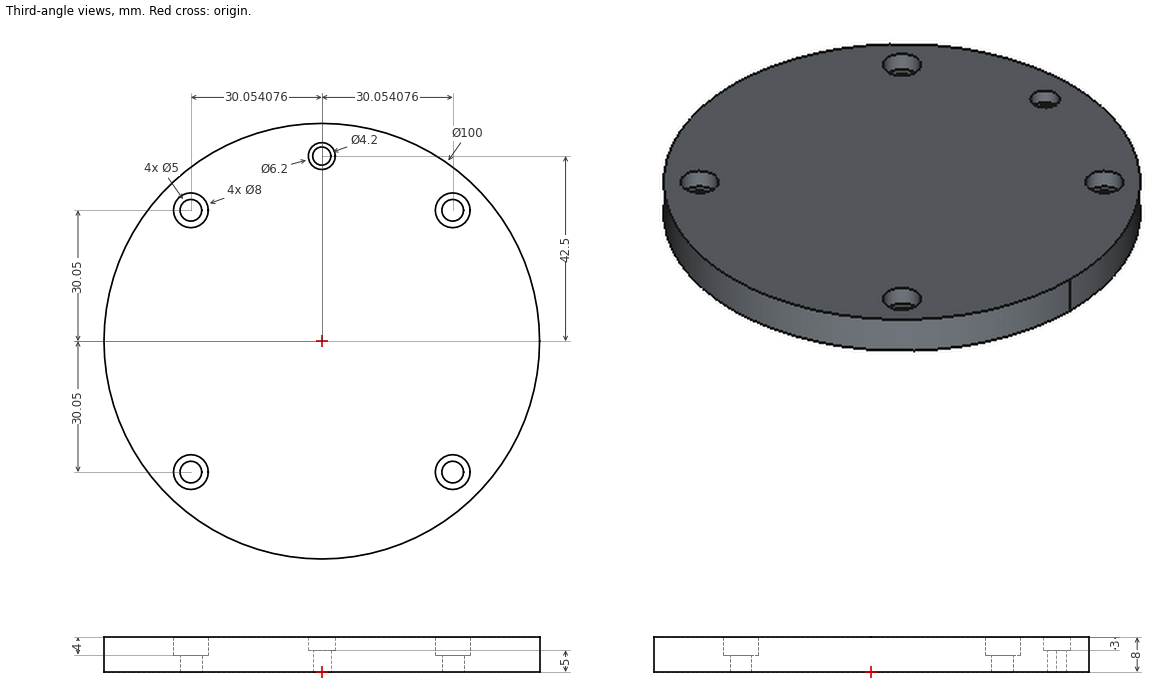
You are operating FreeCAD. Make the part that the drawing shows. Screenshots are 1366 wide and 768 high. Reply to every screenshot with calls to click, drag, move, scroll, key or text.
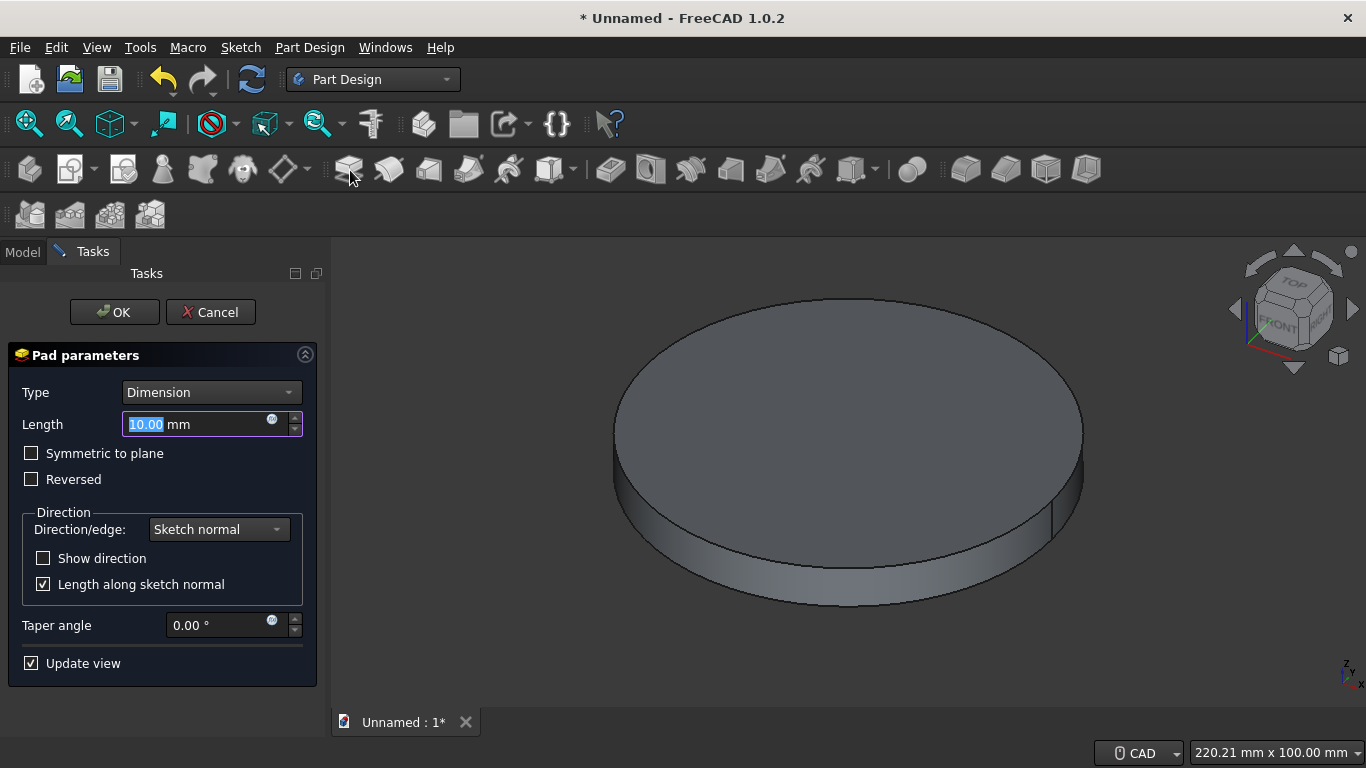
text(8)
key(Tab)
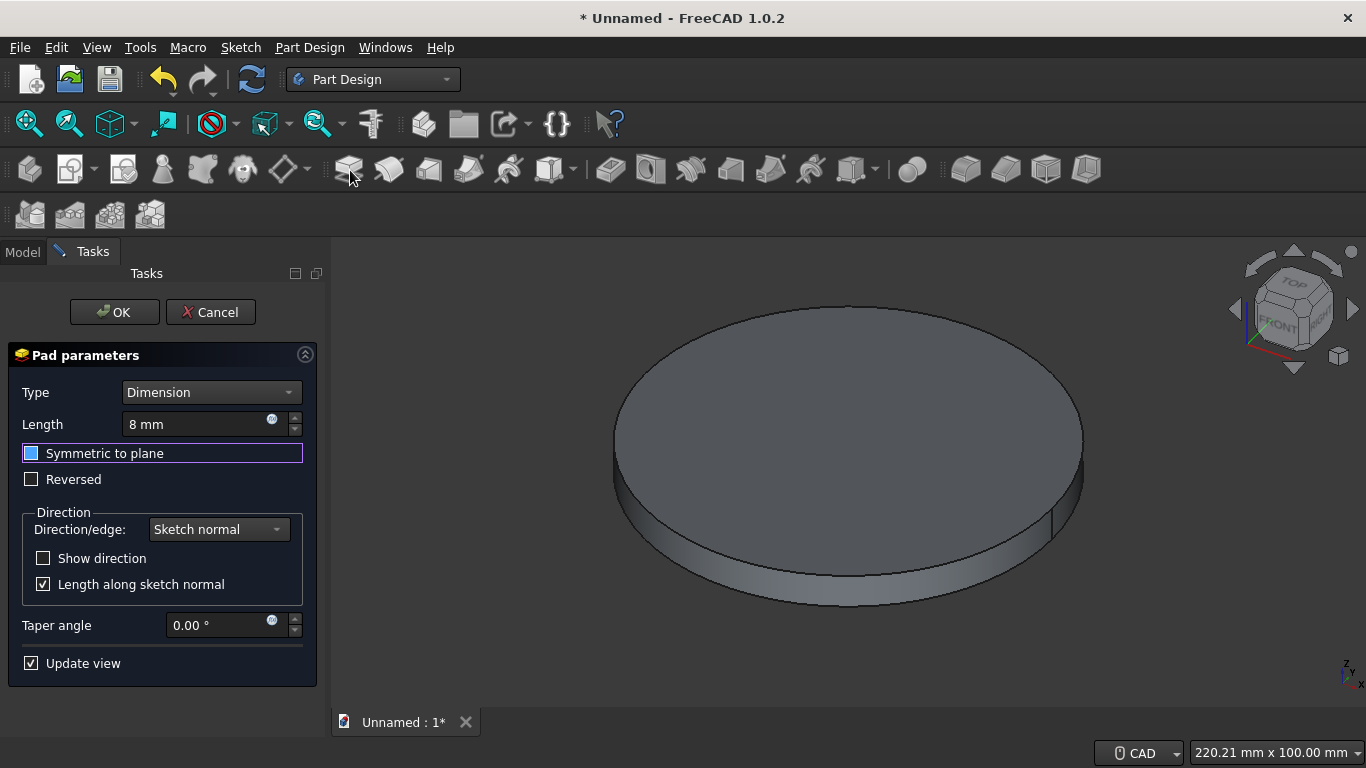
click(115, 312)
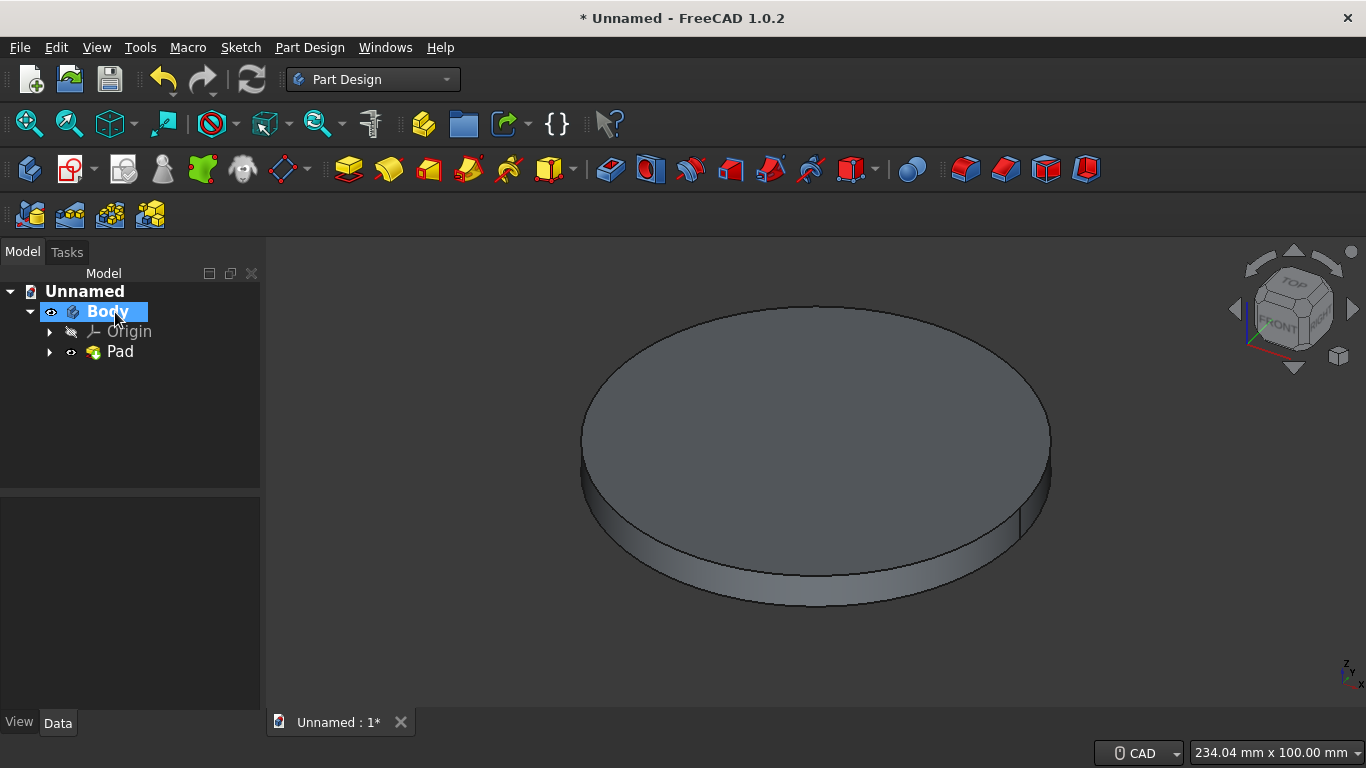
click(816, 440)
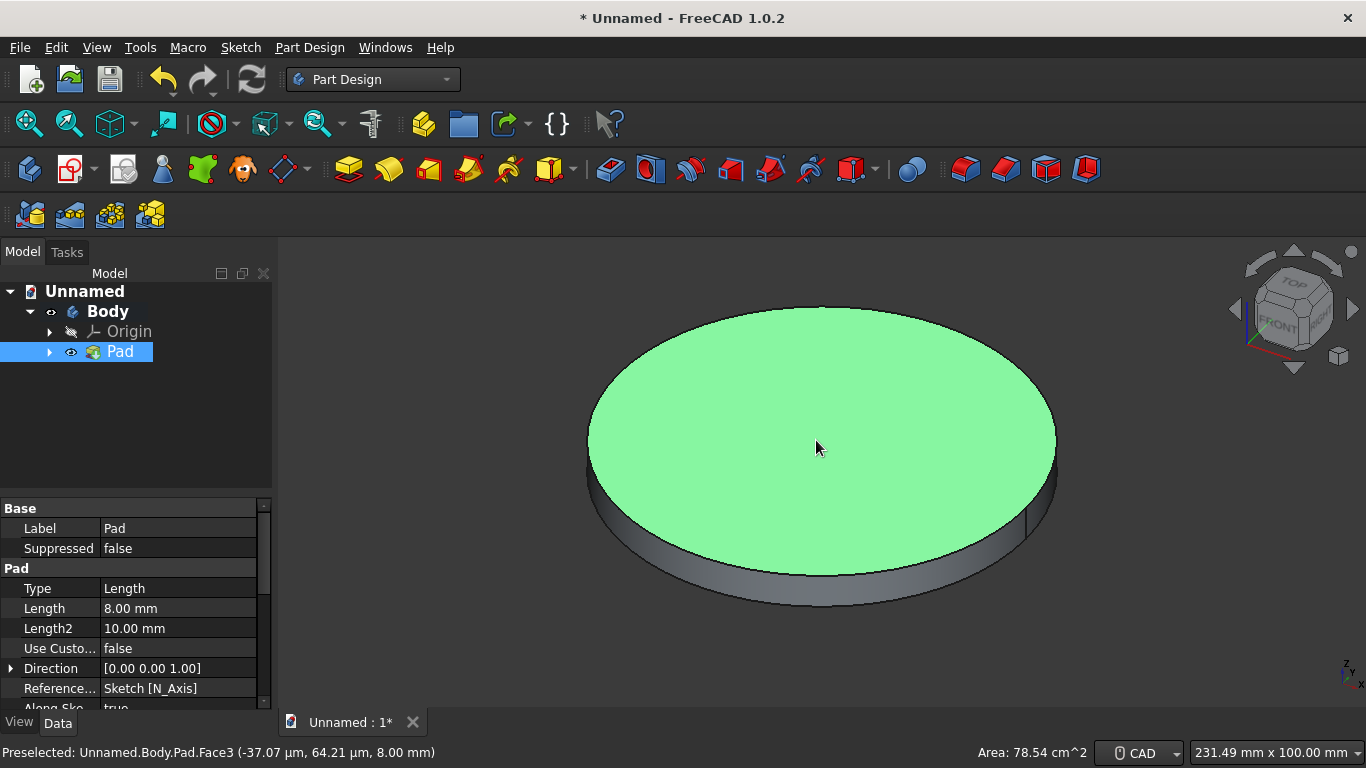
click(70, 170)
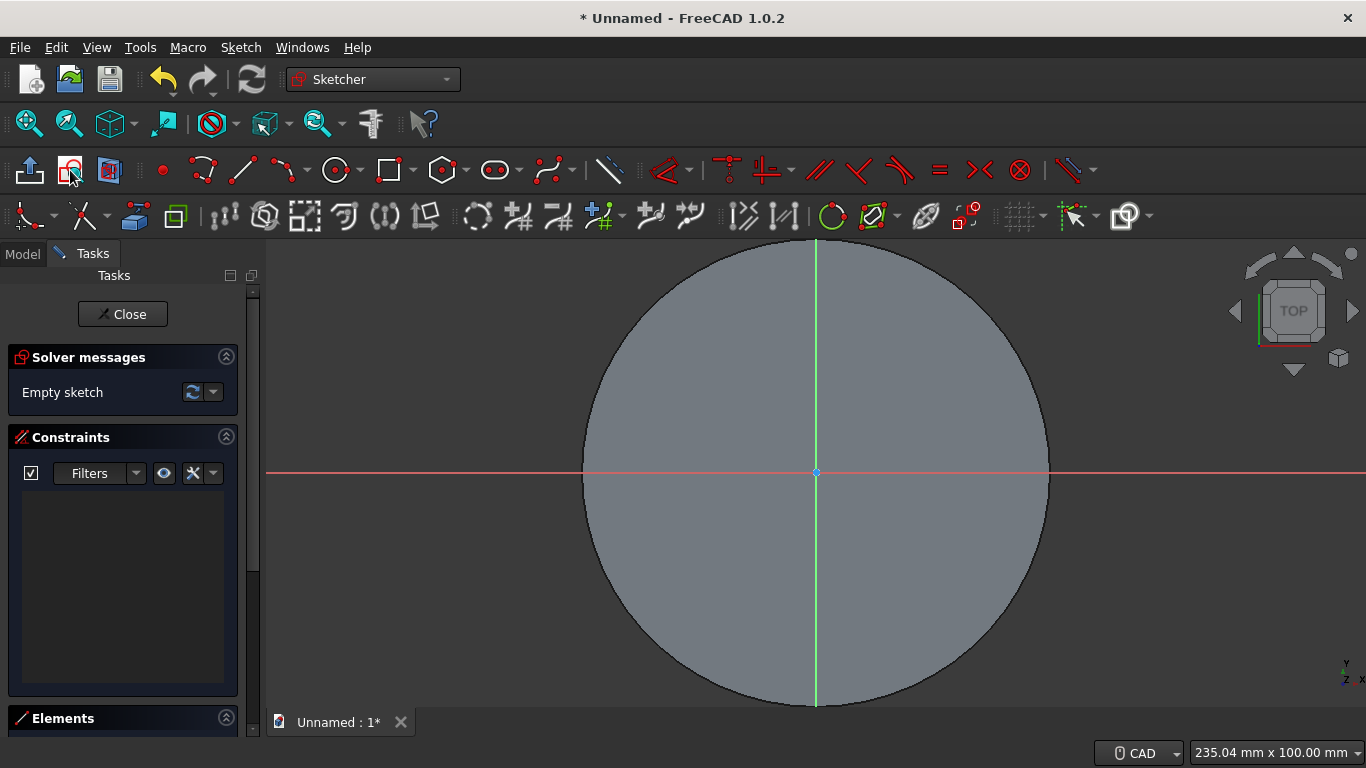
click(336, 170)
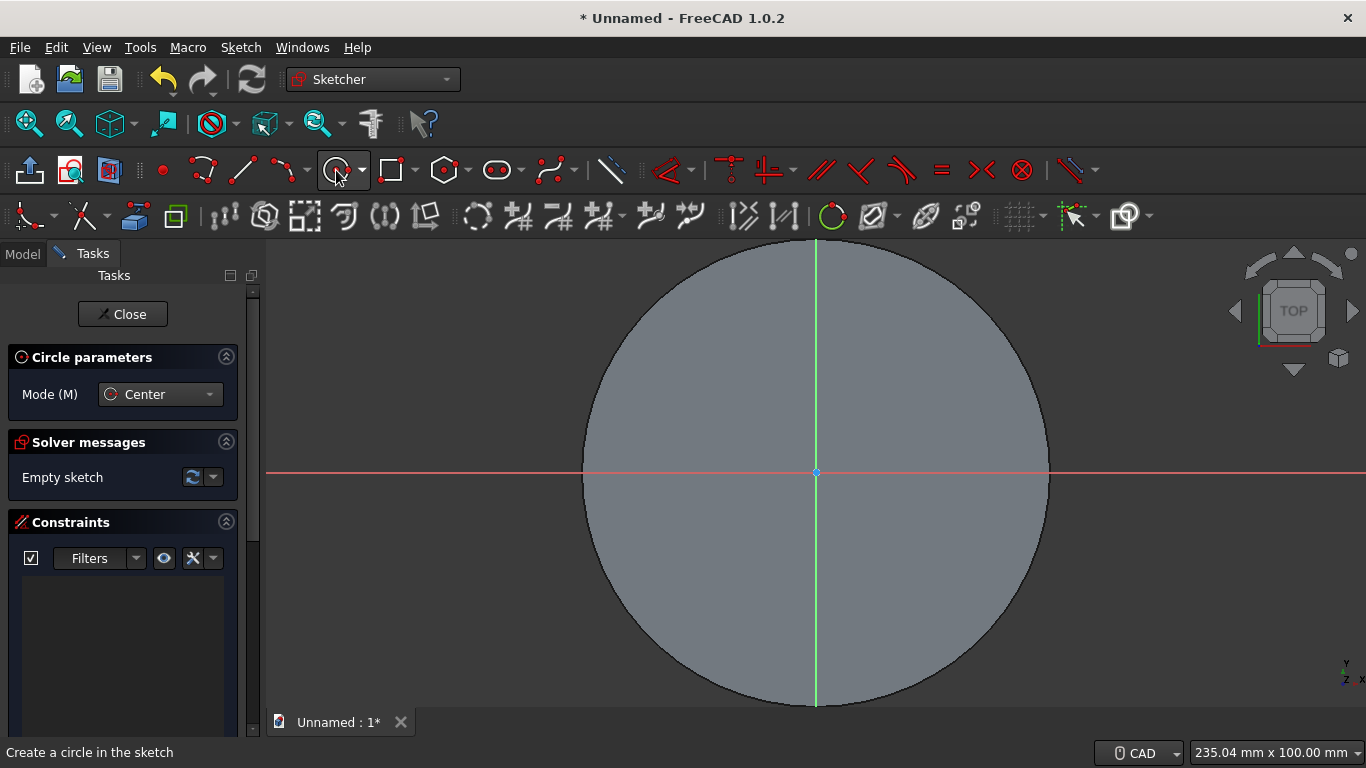
click(675, 332)
move(689, 319)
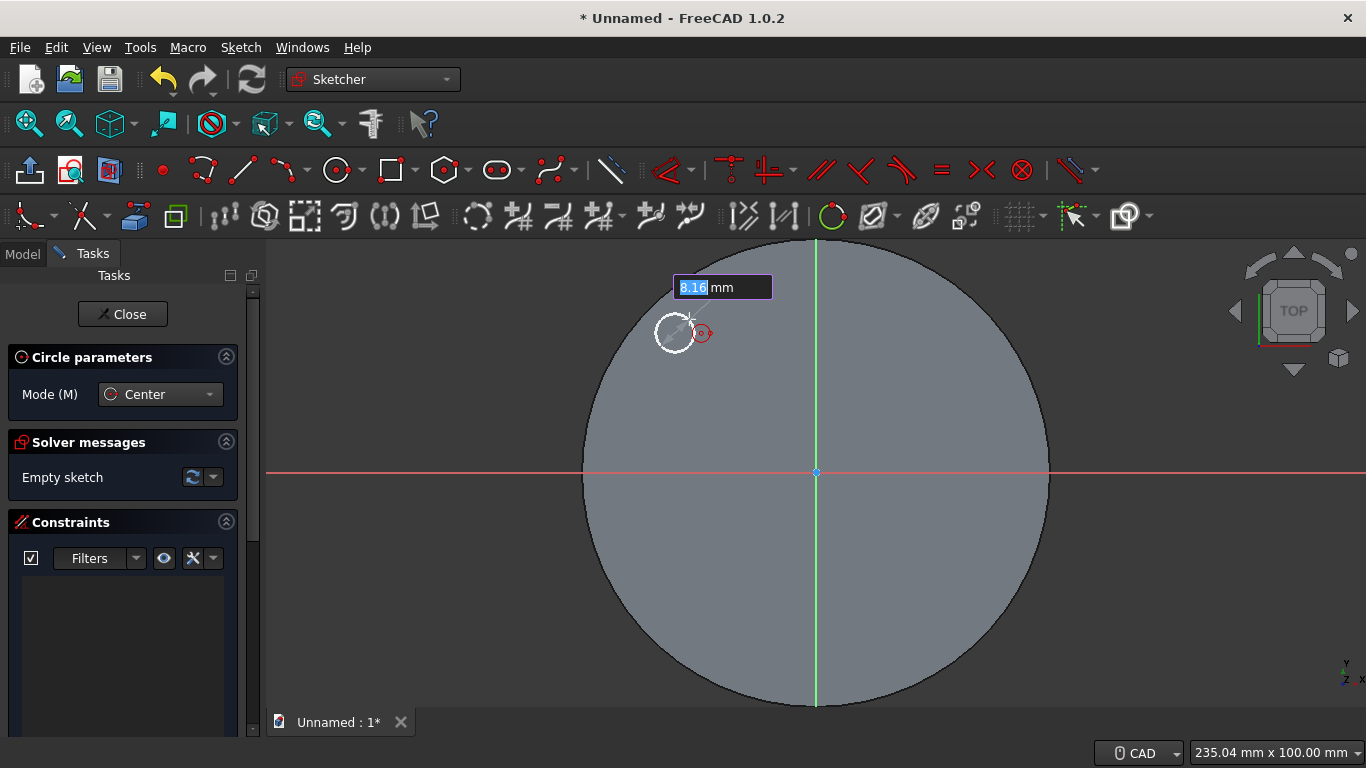
text(8)
key(Return)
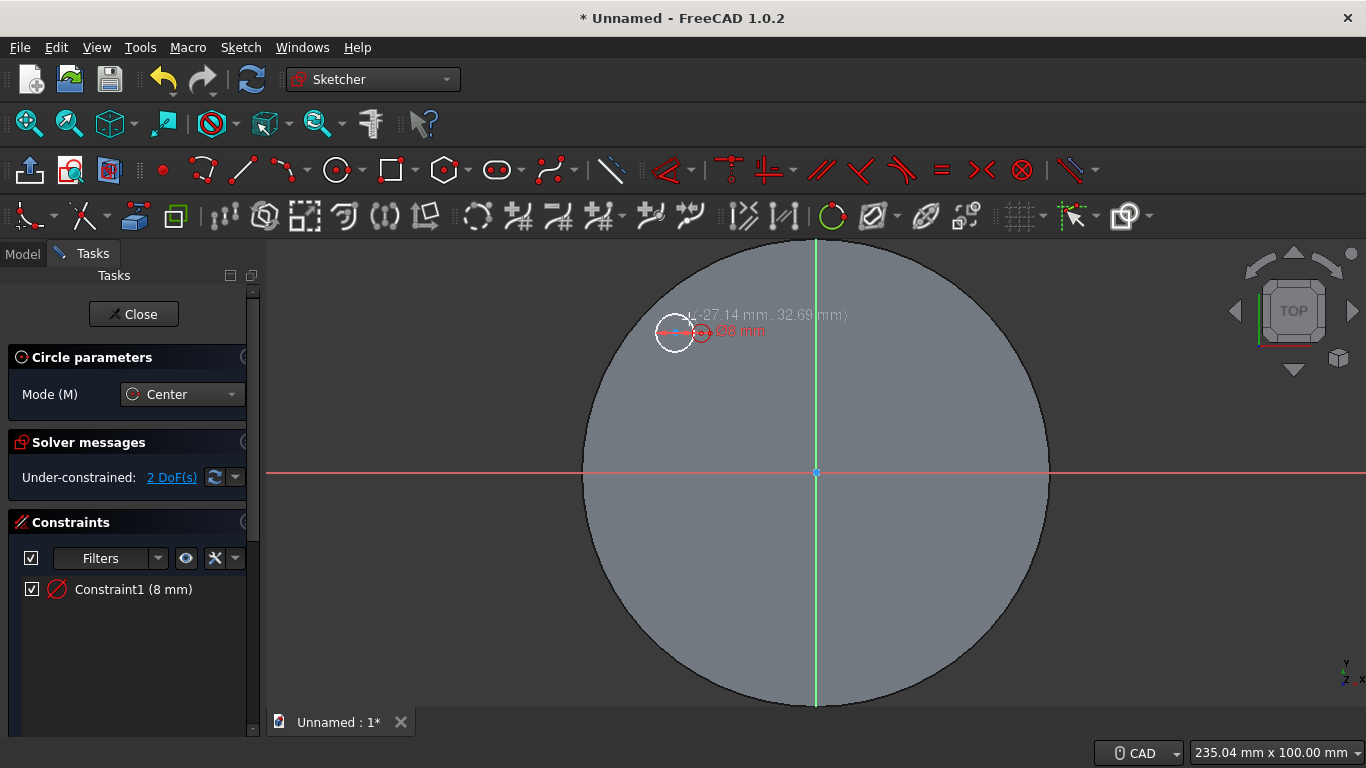
click(957, 332)
move(970, 319)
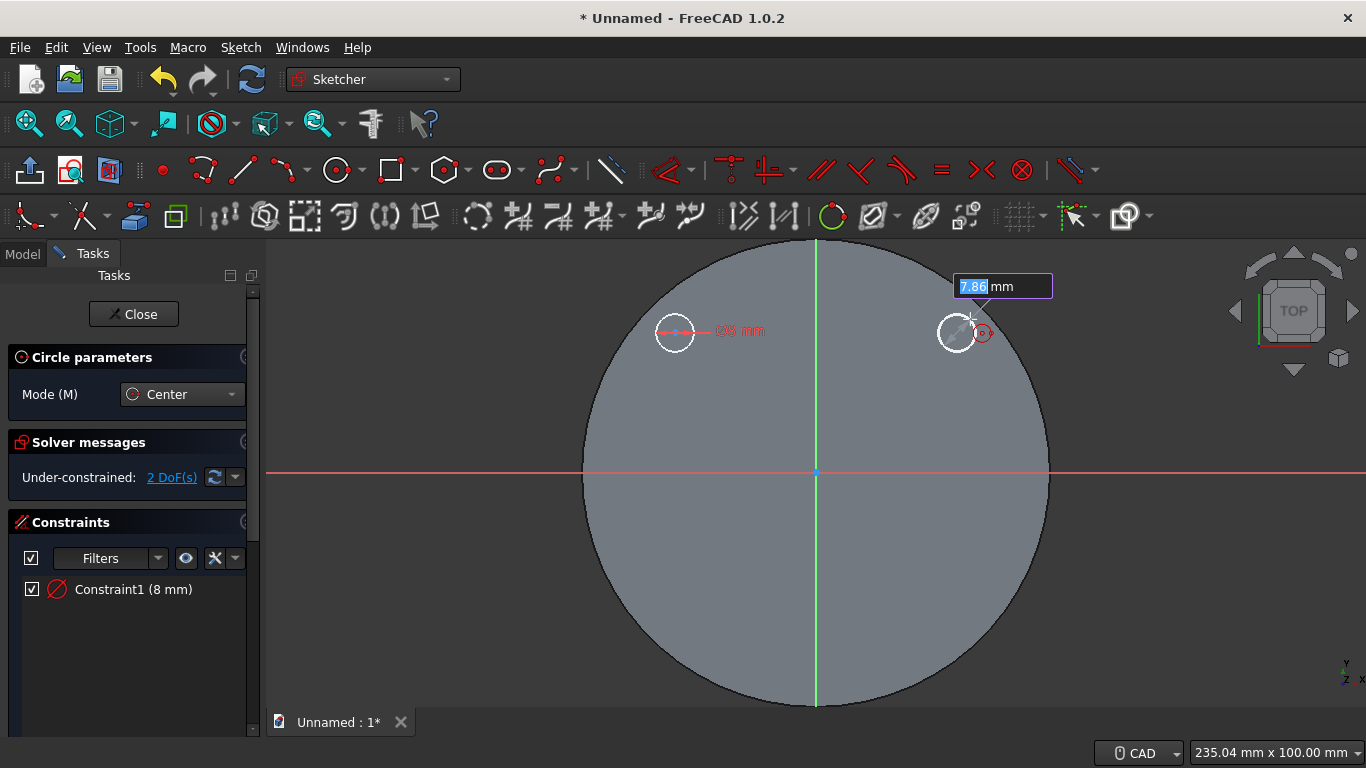
text(8)
key(Return)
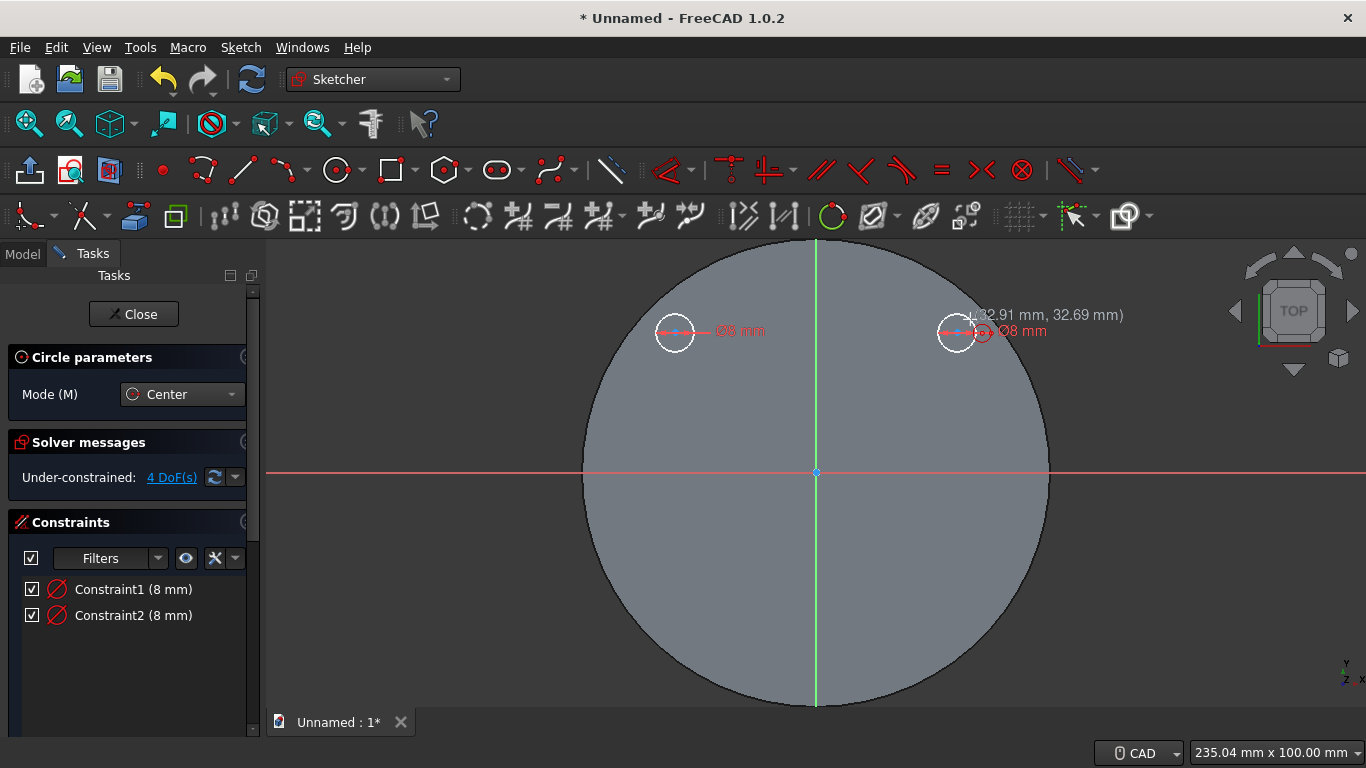
click(675, 614)
move(689, 600)